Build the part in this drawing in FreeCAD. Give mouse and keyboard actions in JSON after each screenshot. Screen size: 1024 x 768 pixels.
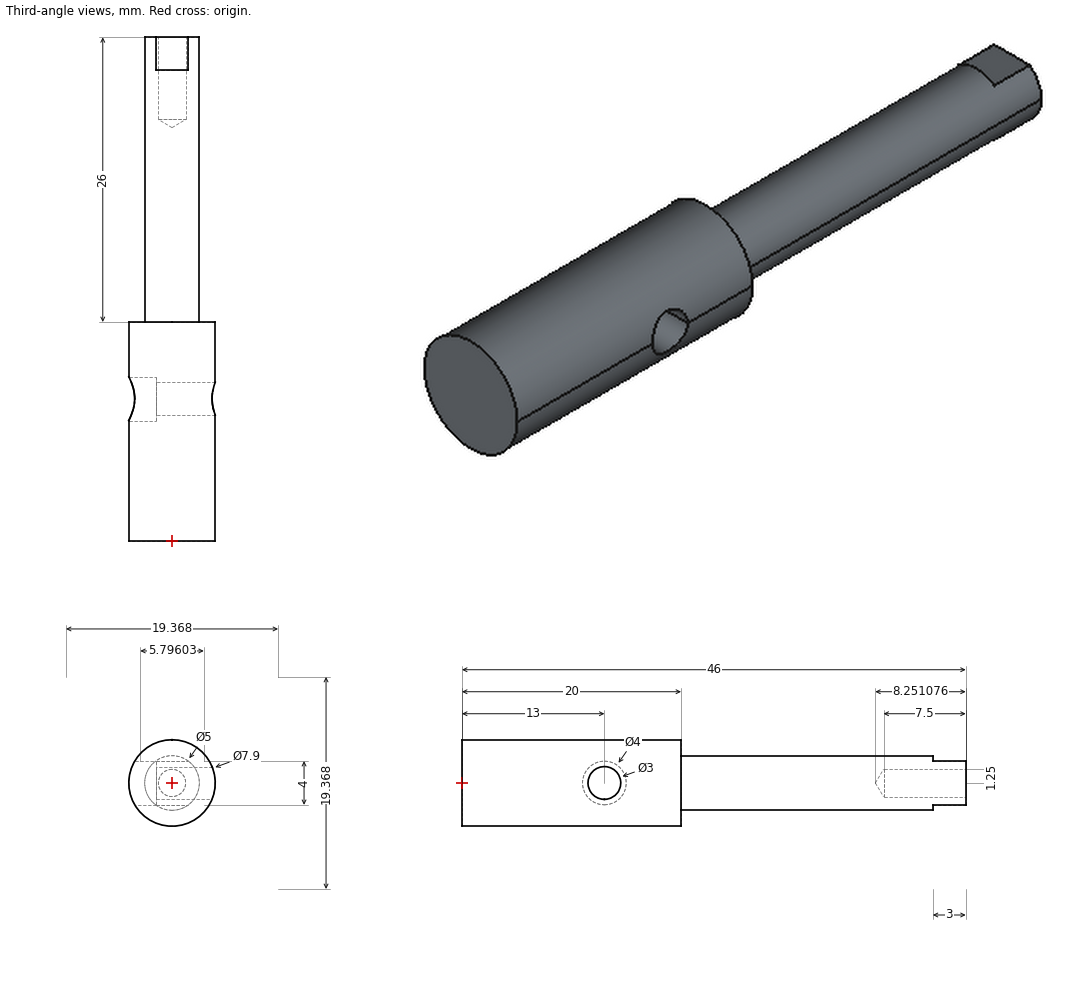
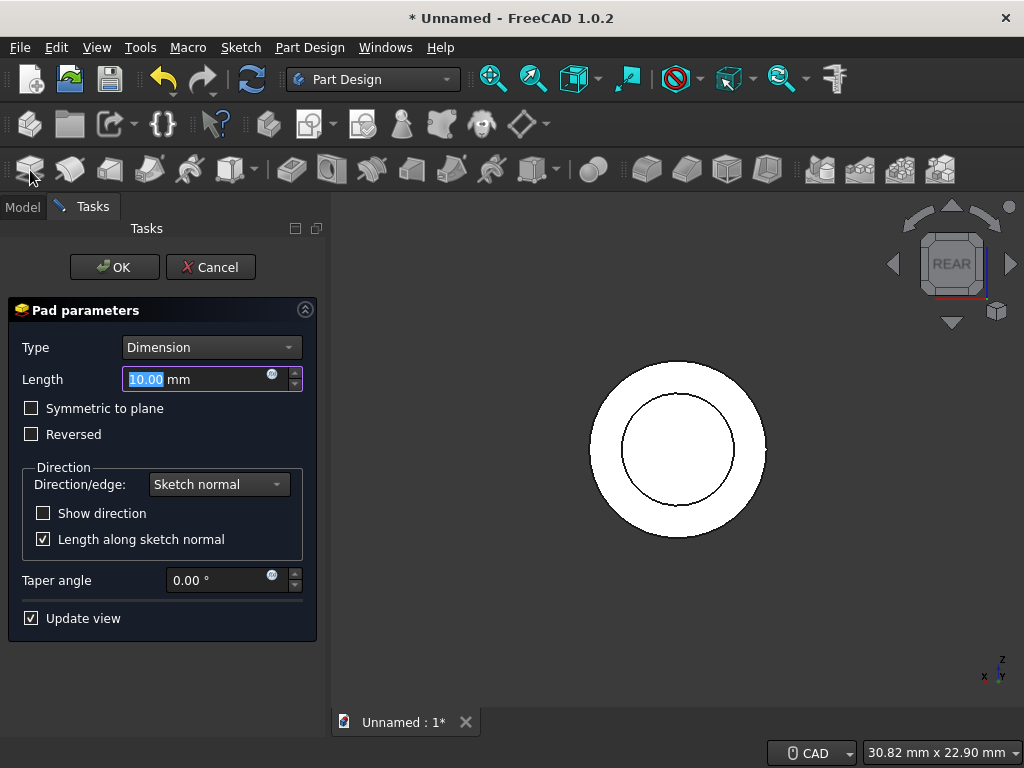
{"action": "type", "text": "26"}
{"action": "key", "text": "Tab"}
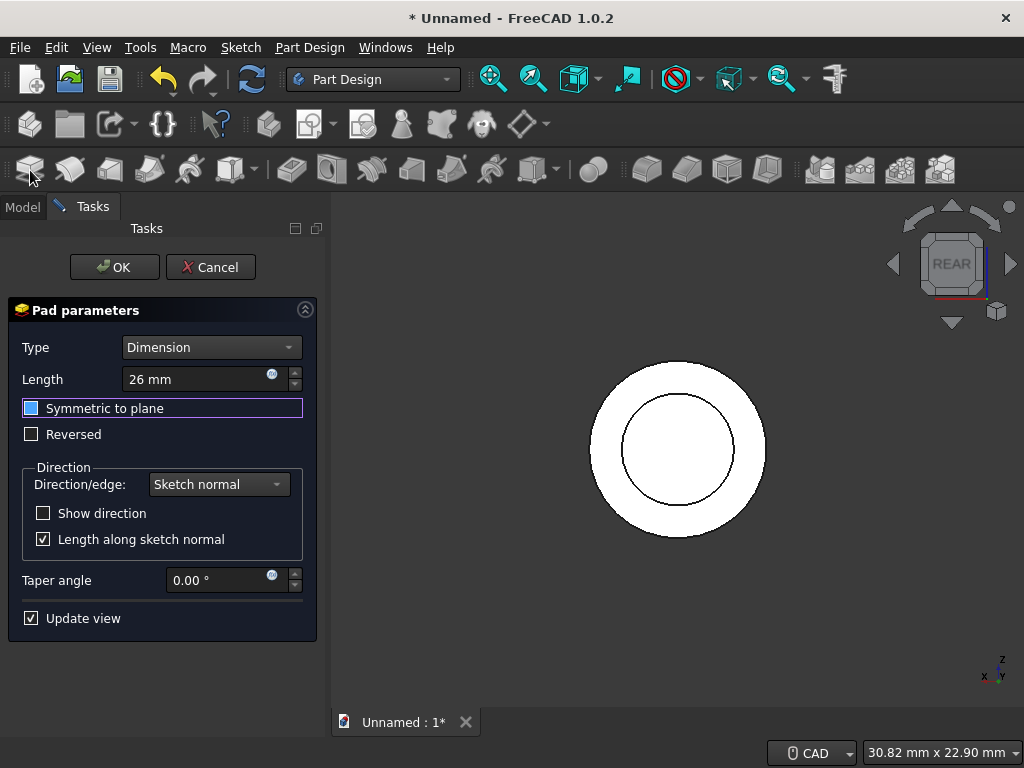
{"action": "left_click", "coordinate": [115, 267]}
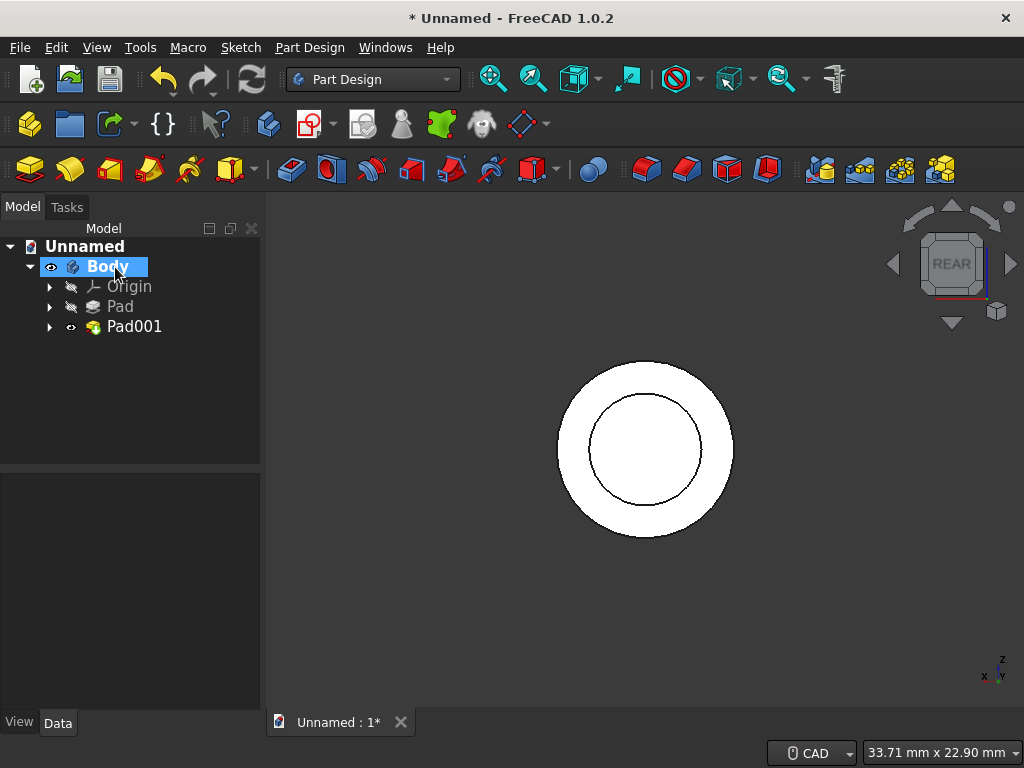
{"action": "left_click", "coordinate": [494, 80]}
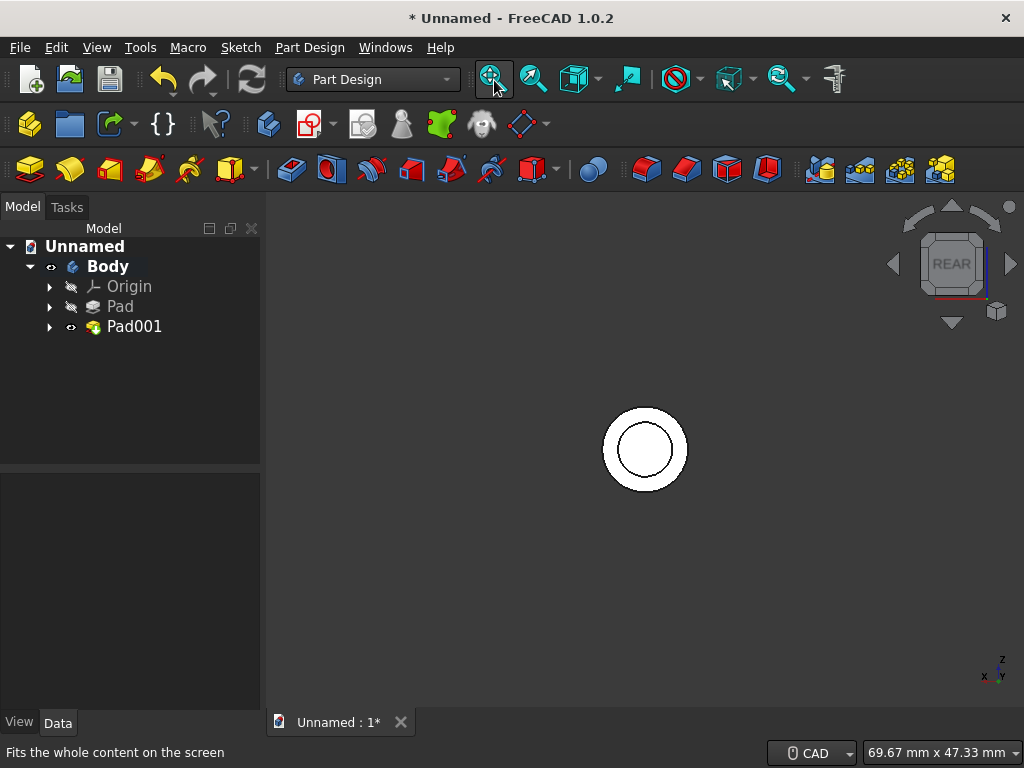
{"action": "left_click", "coordinate": [645, 448]}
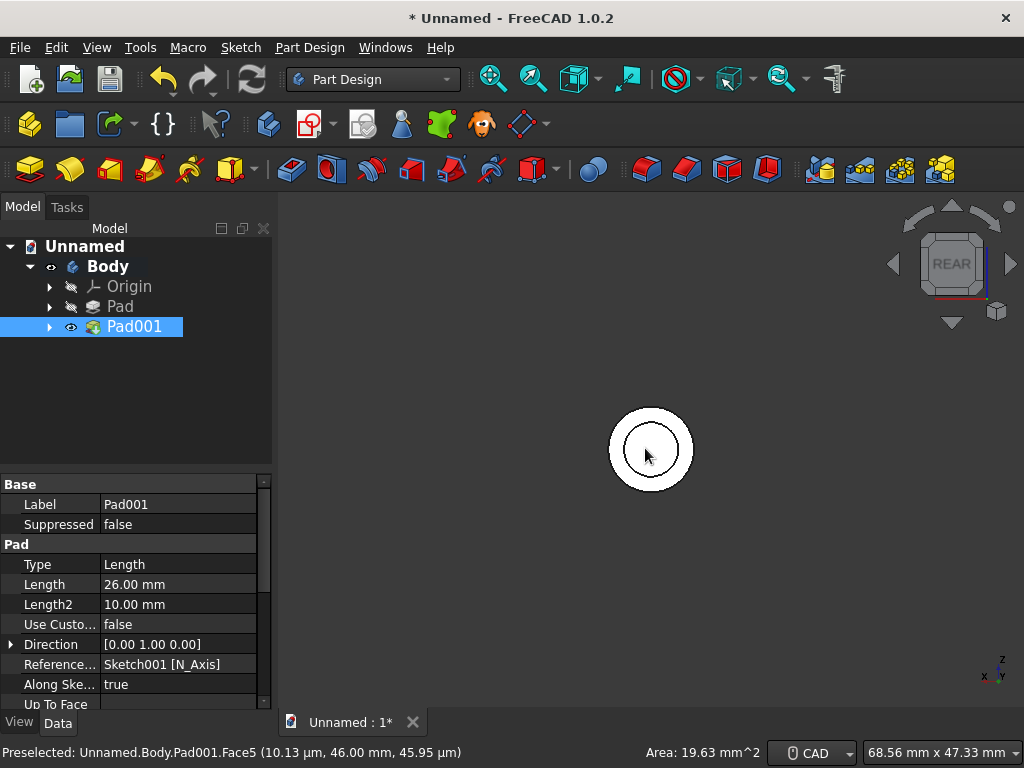
{"action": "left_click", "coordinate": [310, 124]}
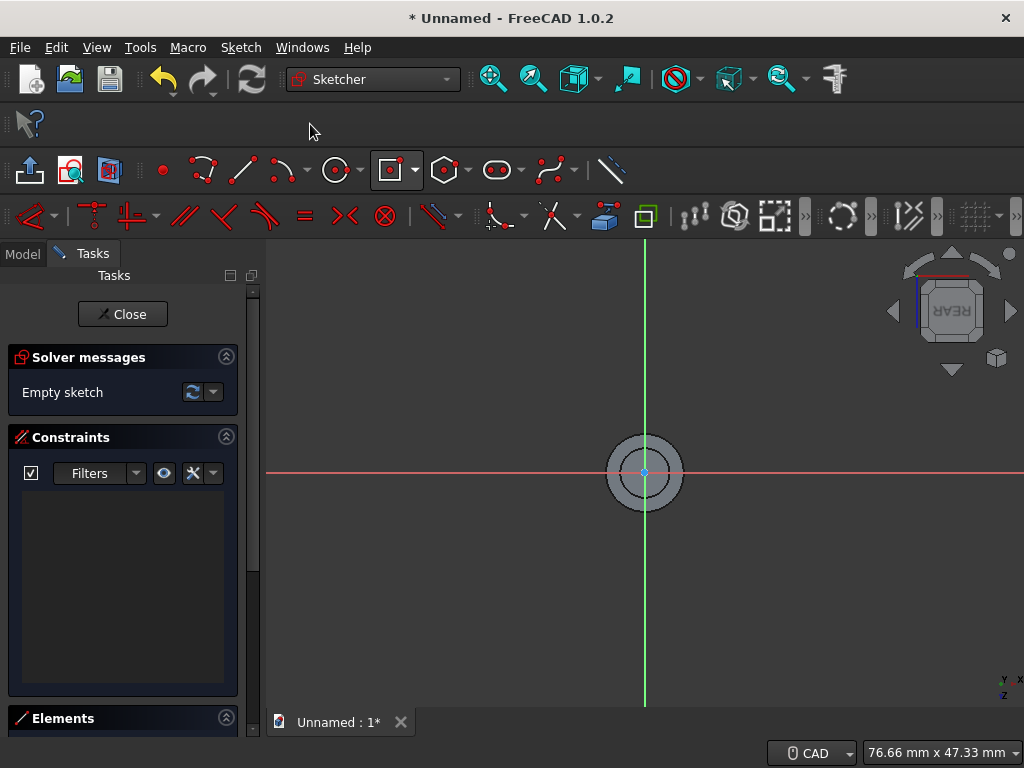
{"action": "scroll", "coordinate": [784, 473], "scroll_direction": "up", "scroll_amount": 2}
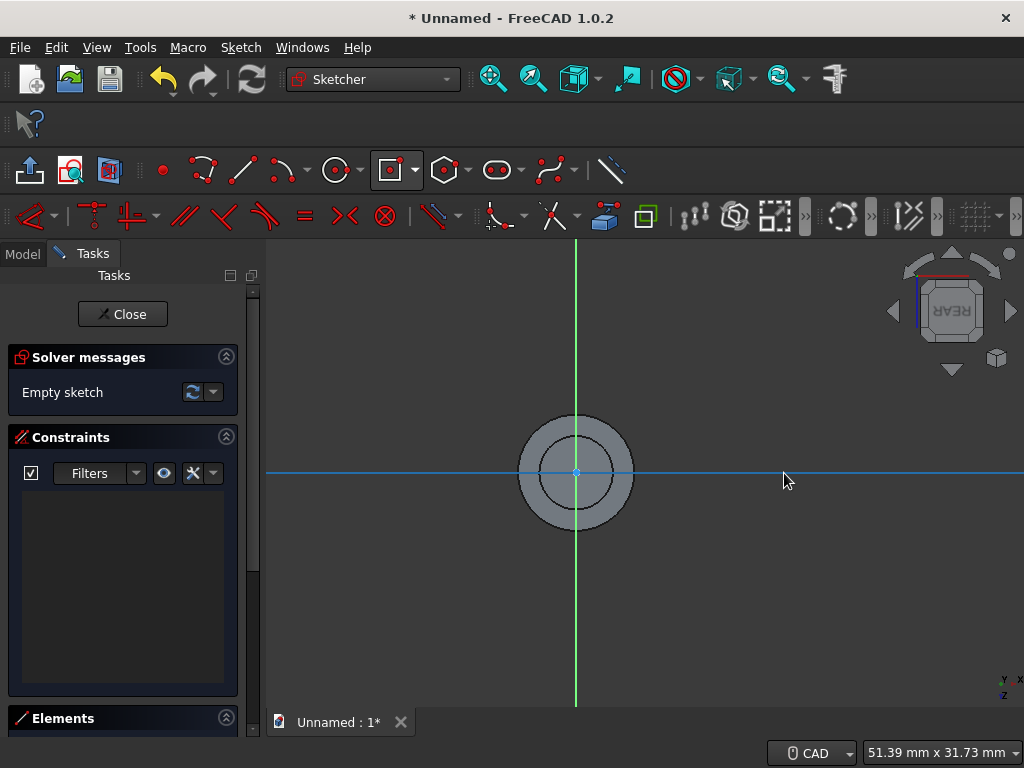
{"action": "left_click", "coordinate": [390, 170]}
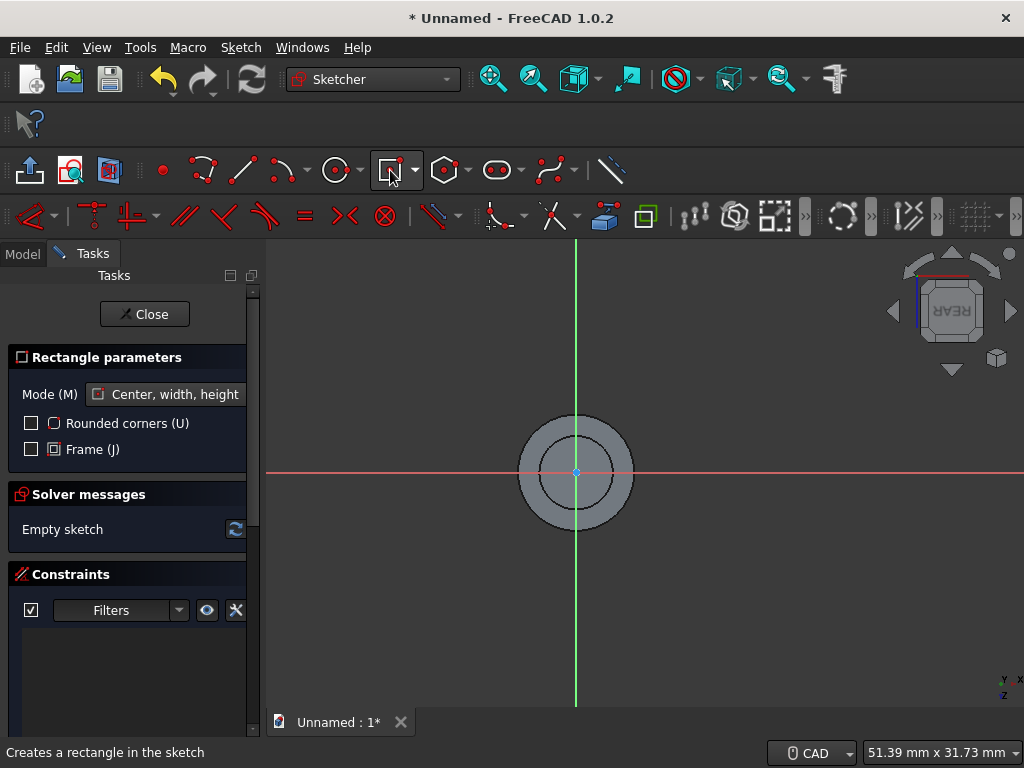
{"action": "left_click", "coordinate": [576, 473]}
{"action": "mouse_move", "coordinate": [719, 330]}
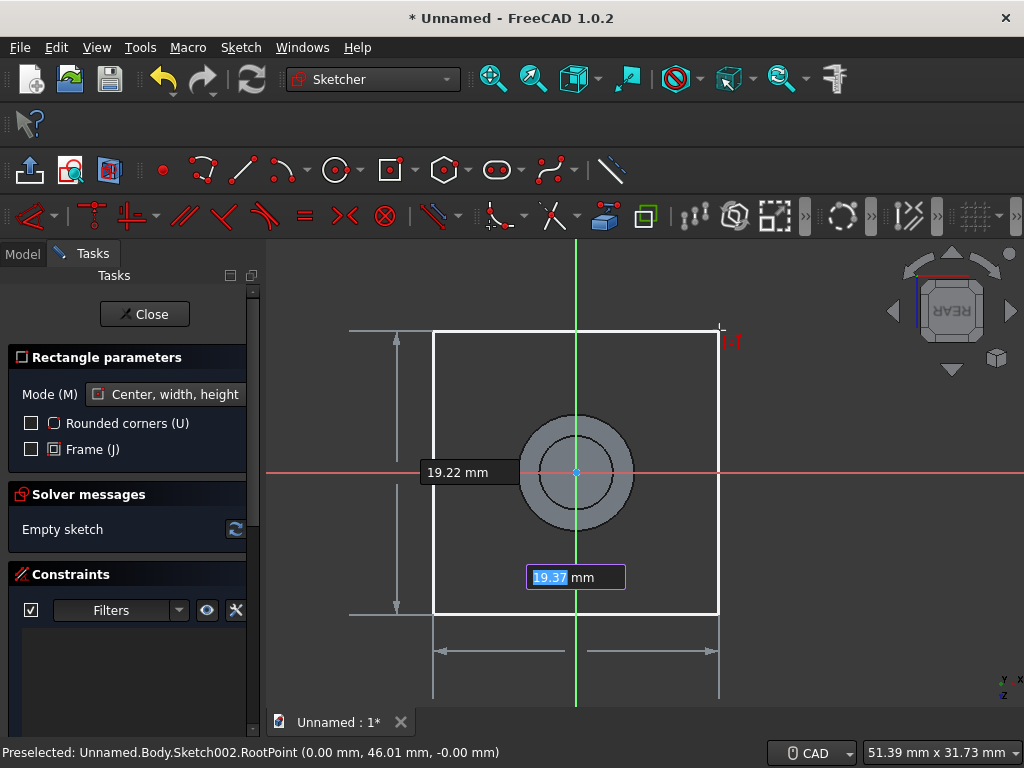
{"action": "type", "text": "19.368"}
{"action": "key", "text": "Tab"}
{"action": "type", "text": "19.368"}
{"action": "key", "text": "Return"}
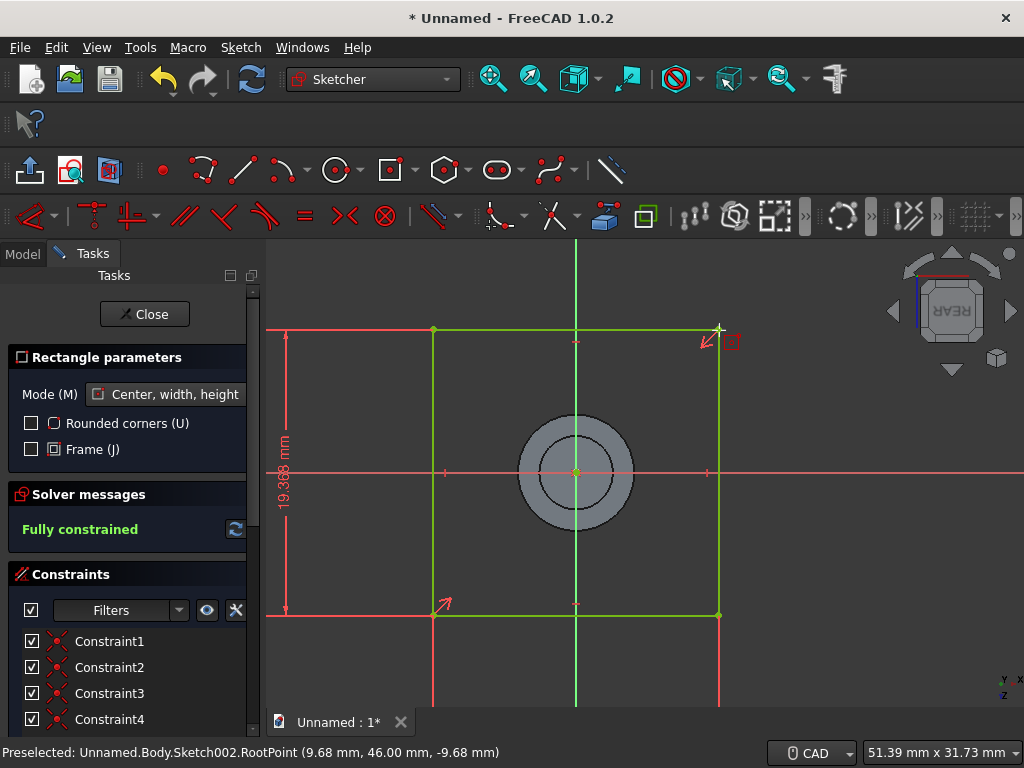
{"action": "left_click", "coordinate": [576, 473]}
{"action": "mouse_move", "coordinate": [619, 443]}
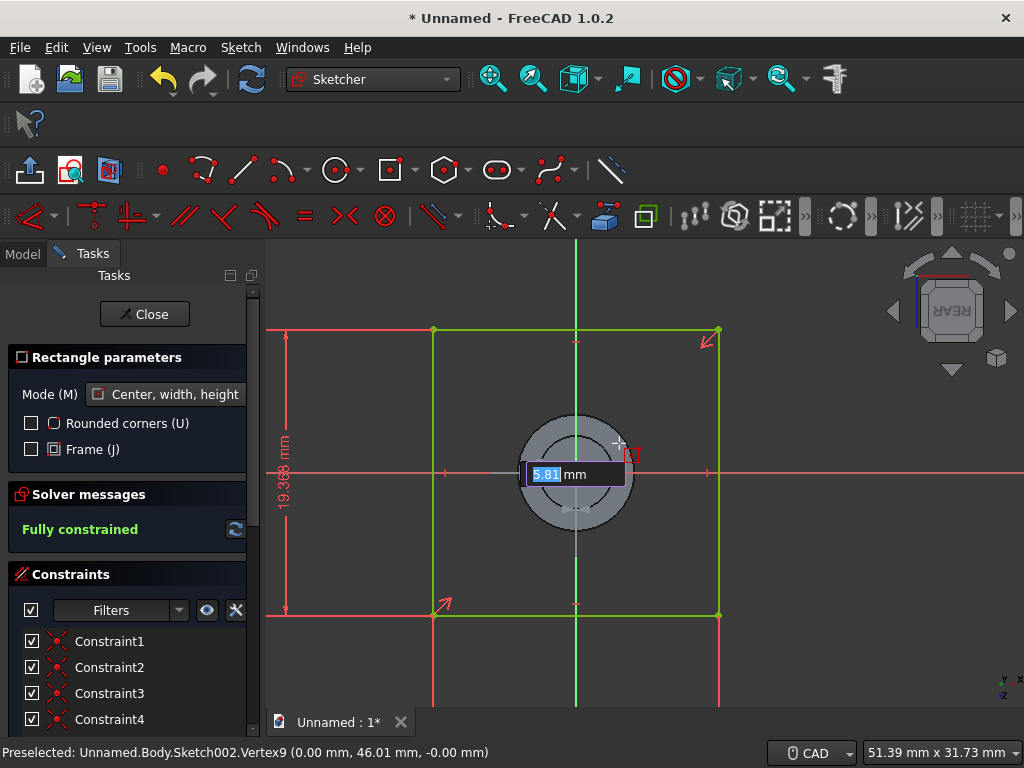
{"action": "type", "text": "5.79603"}
{"action": "key", "text": "Tab"}
{"action": "type", "text": "4"}
{"action": "key", "text": "Return"}
{"action": "key", "text": "Escape"}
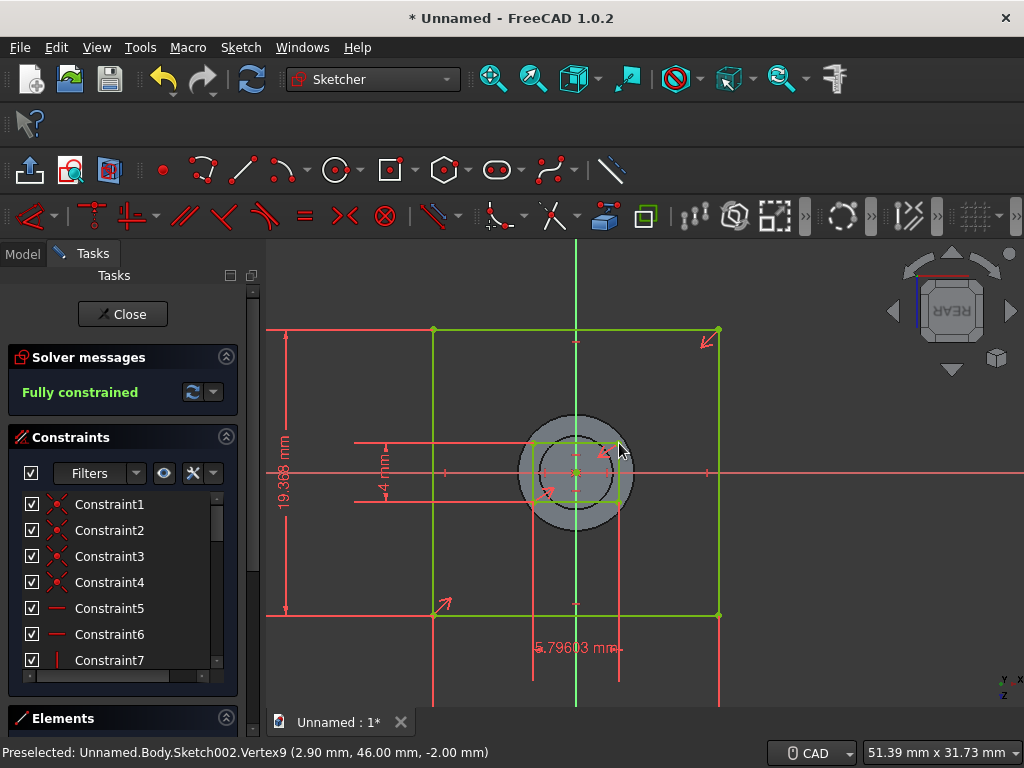
{"action": "left_click", "coordinate": [123, 314]}